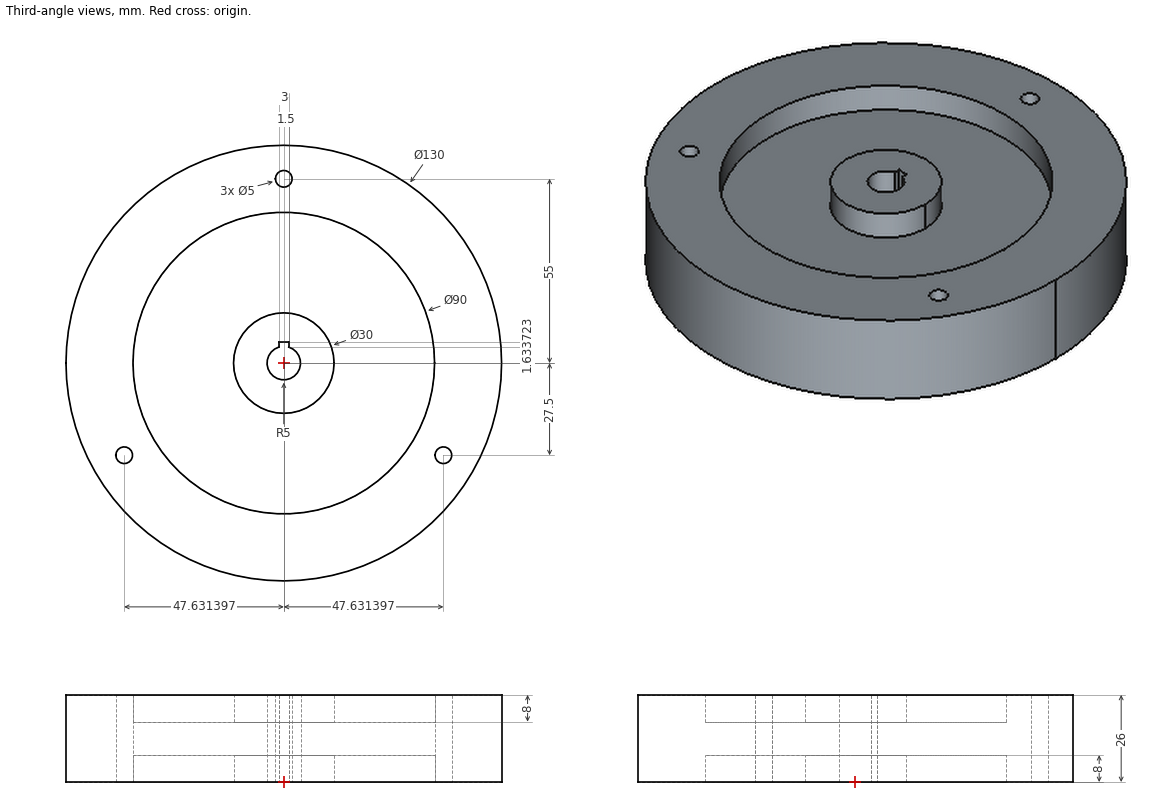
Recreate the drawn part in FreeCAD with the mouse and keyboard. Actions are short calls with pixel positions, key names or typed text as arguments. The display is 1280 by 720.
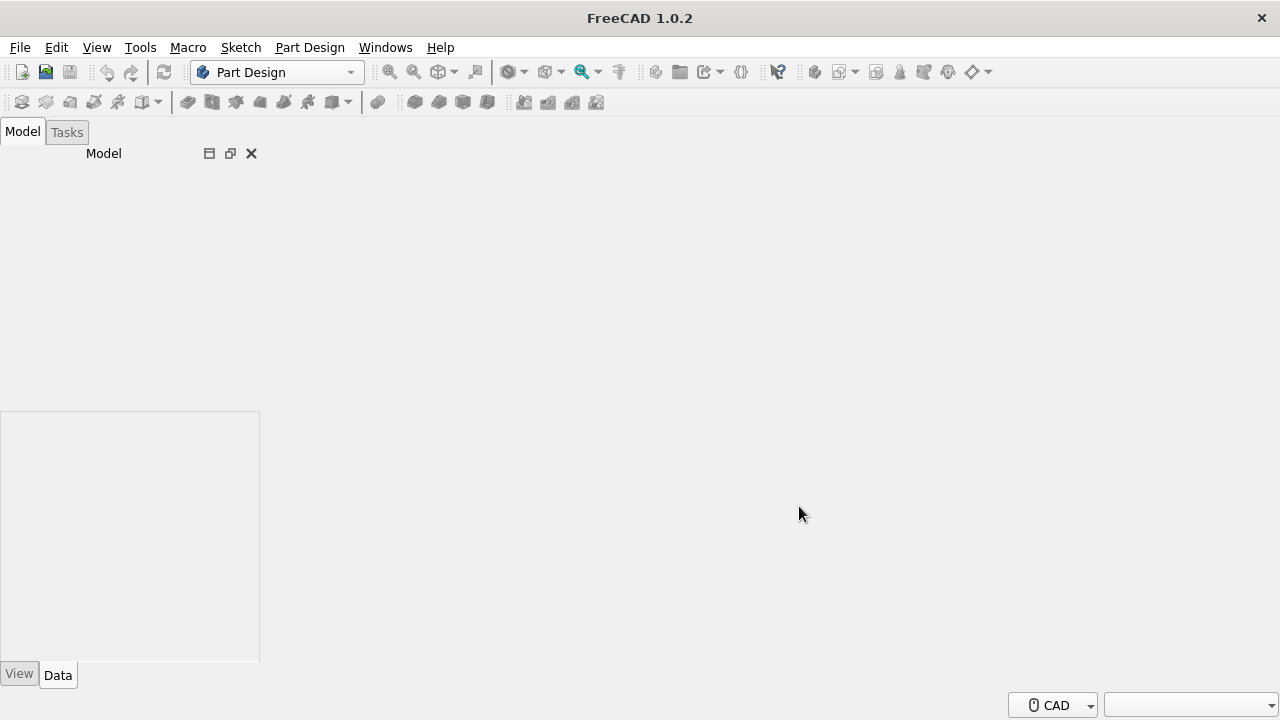
key(ctrl+n)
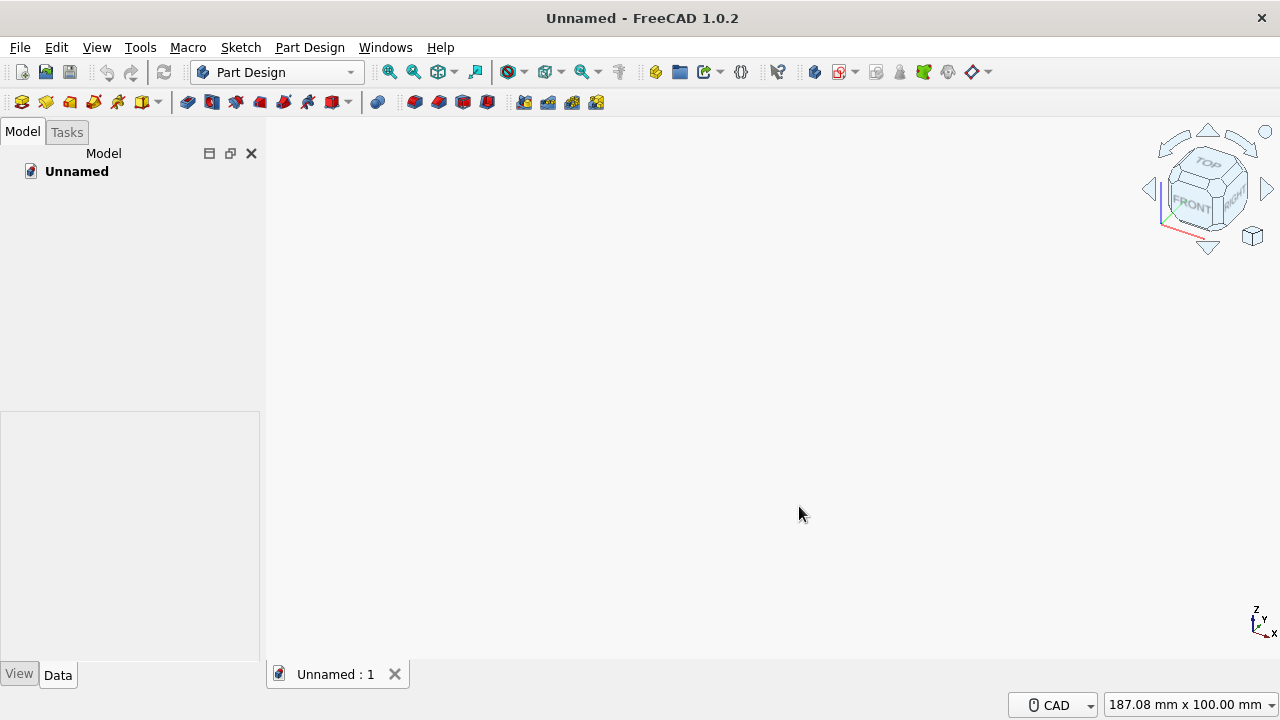
click(840, 72)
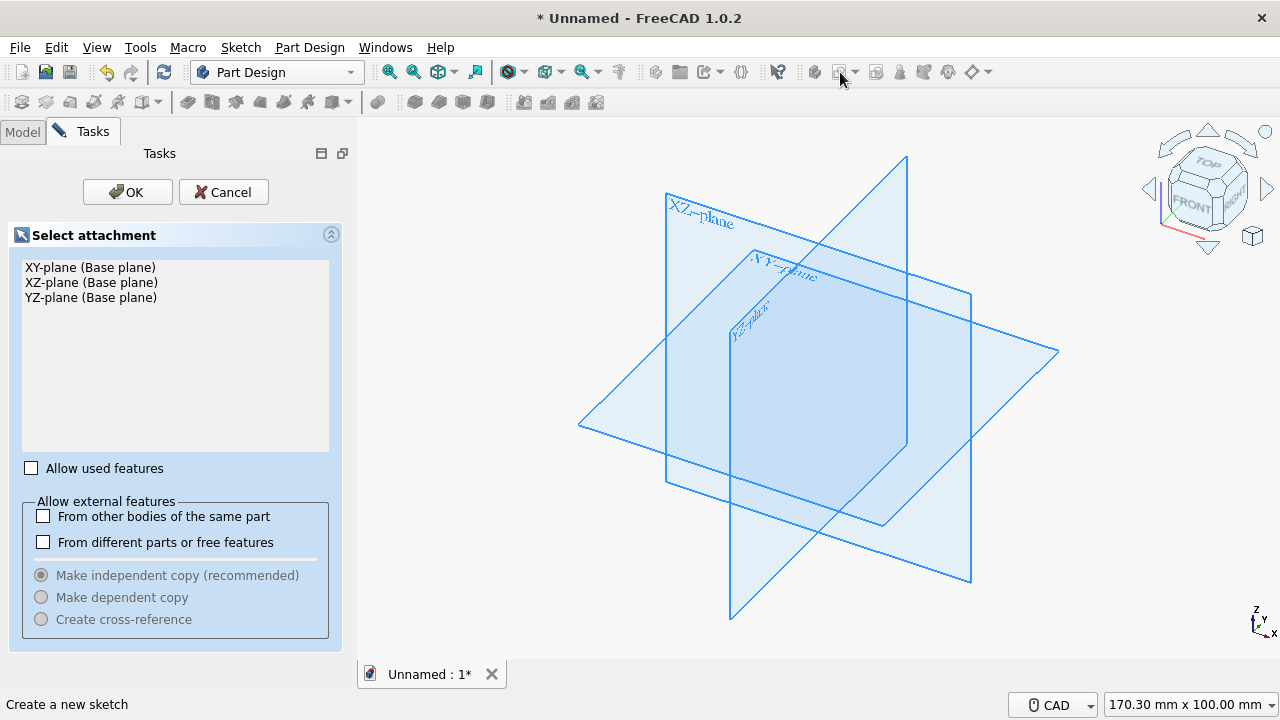
click(82, 268)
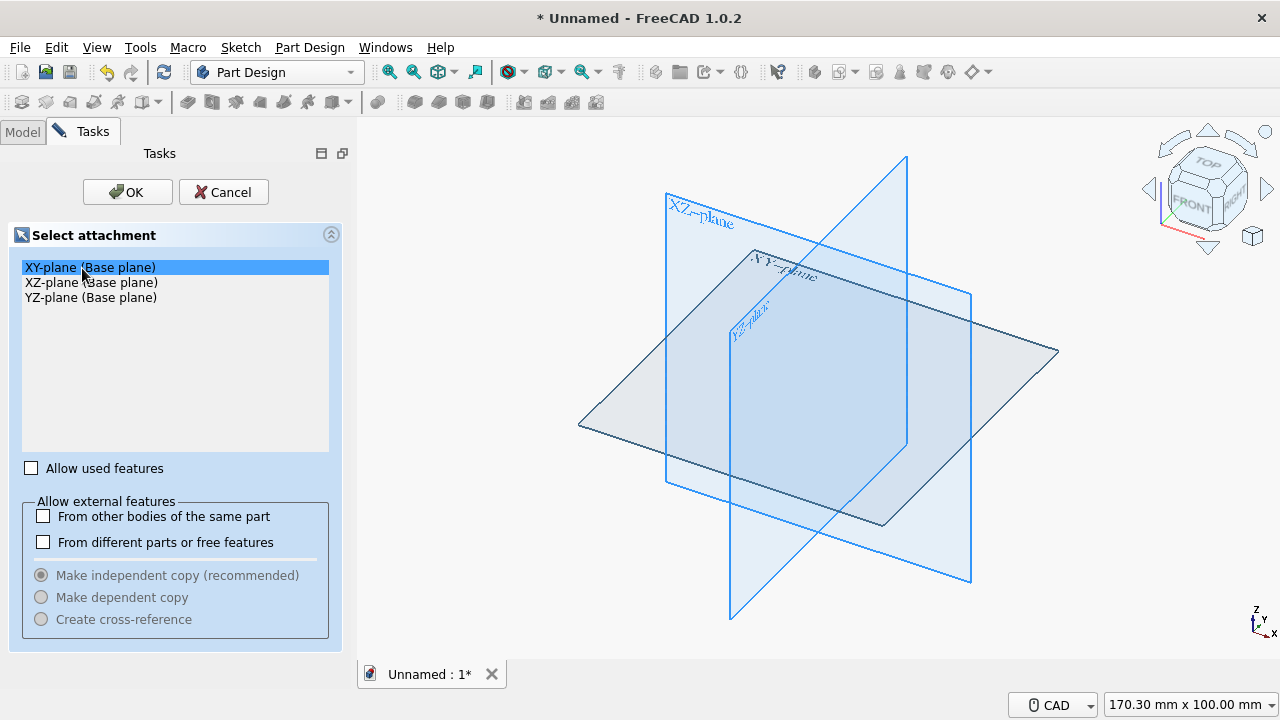
click(128, 192)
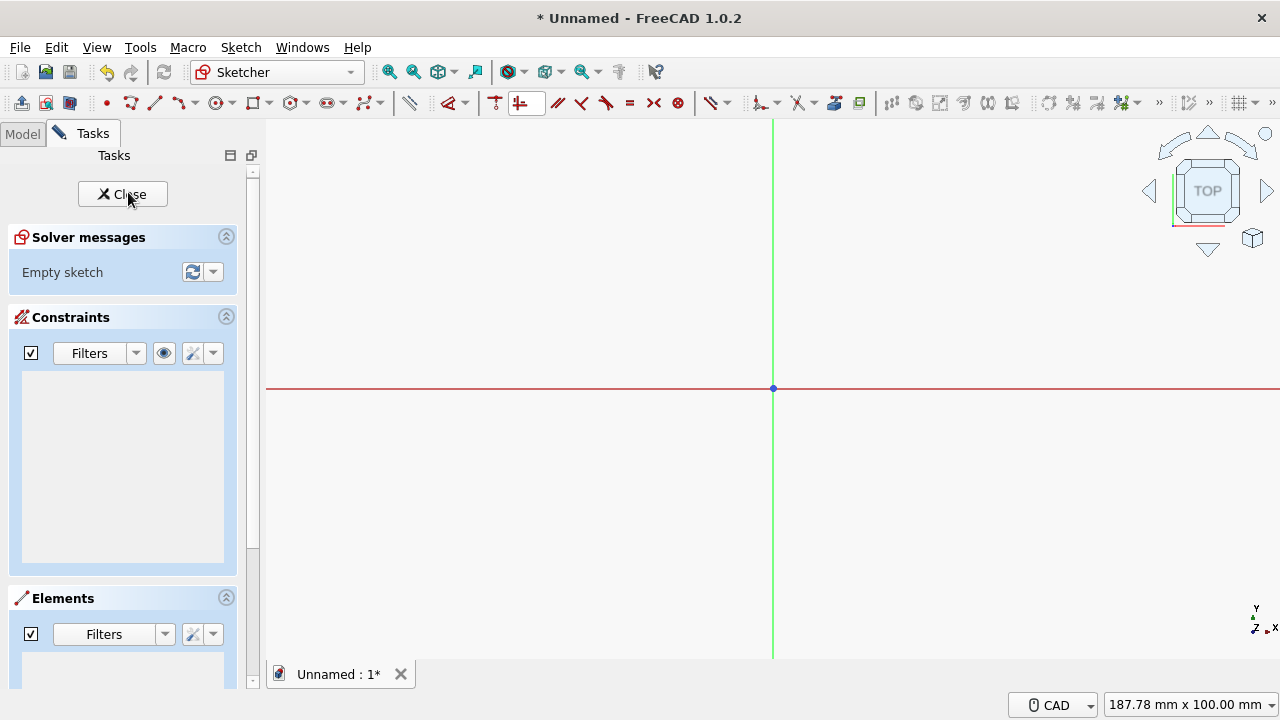
scroll(649, 389, down, 4)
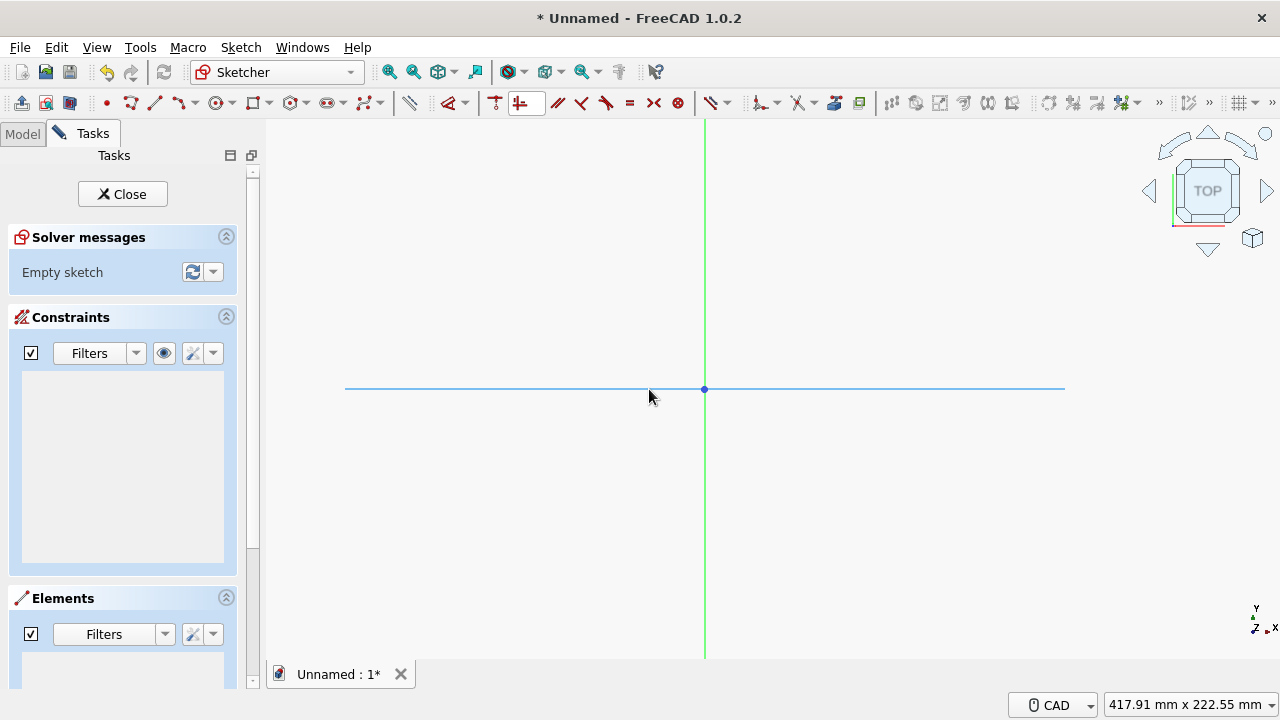
key(g)
key(c)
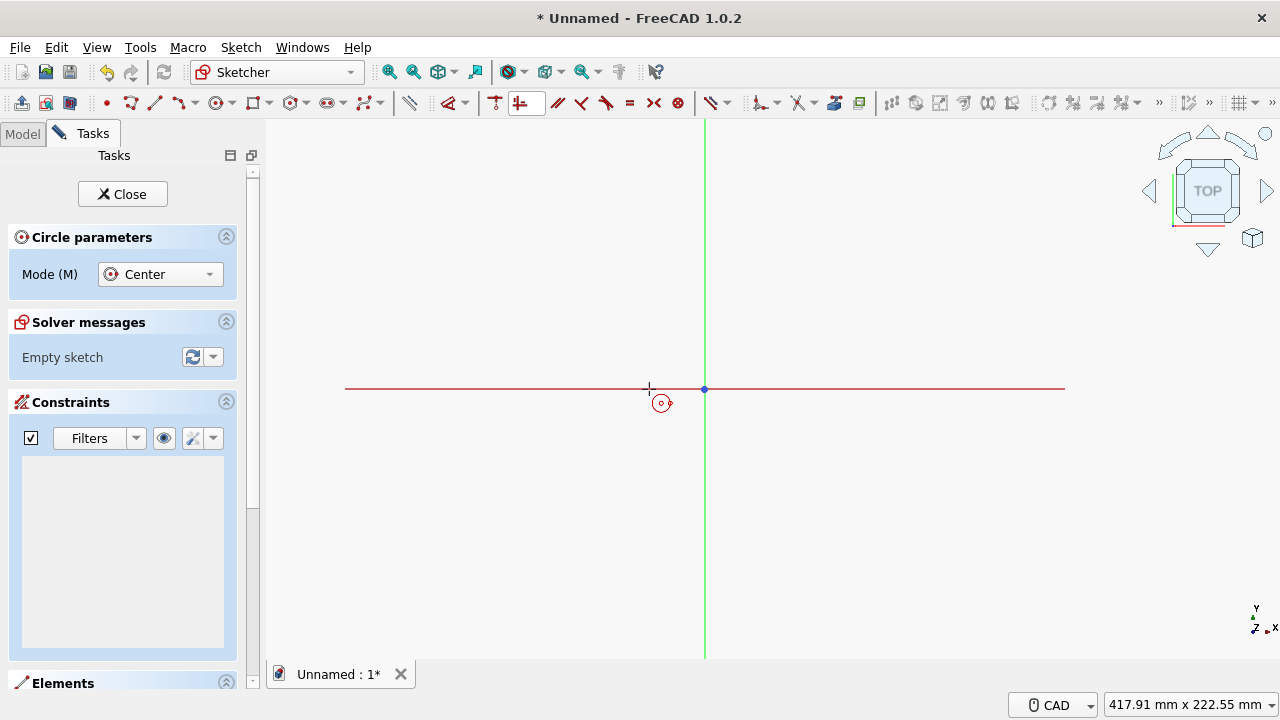
click(705, 389)
click(816, 278)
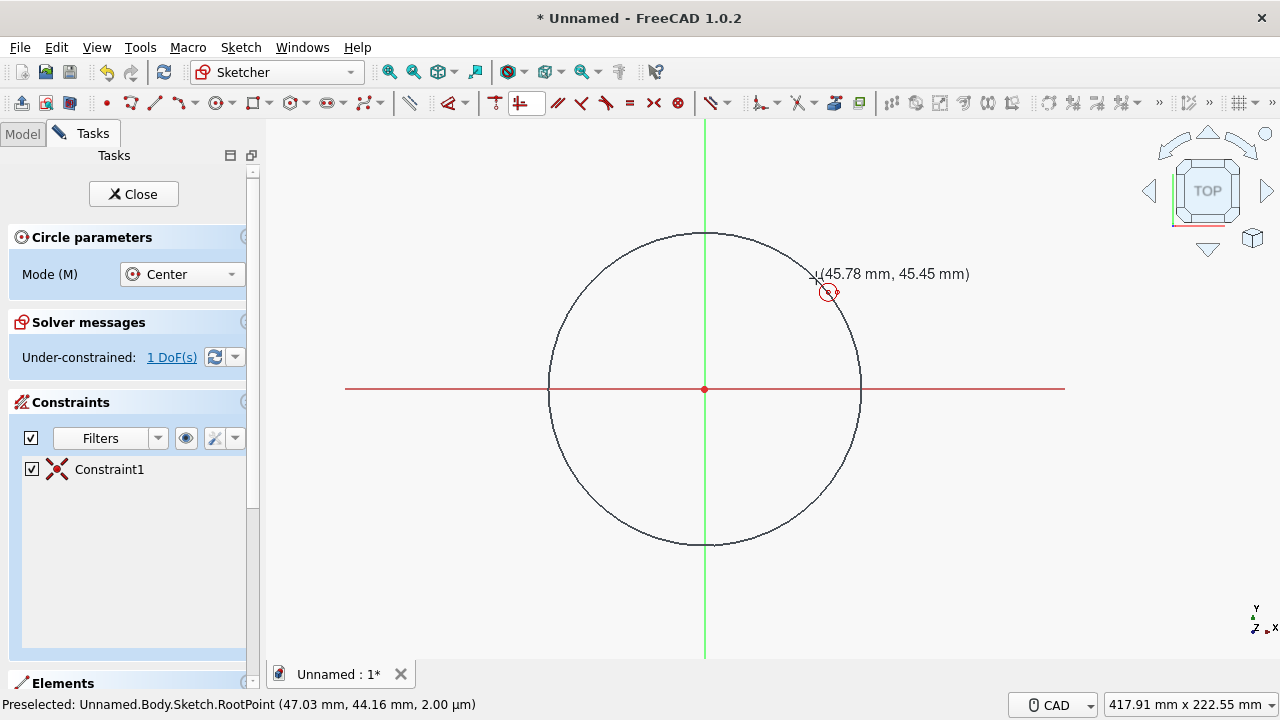
scroll(705, 256, up, 7)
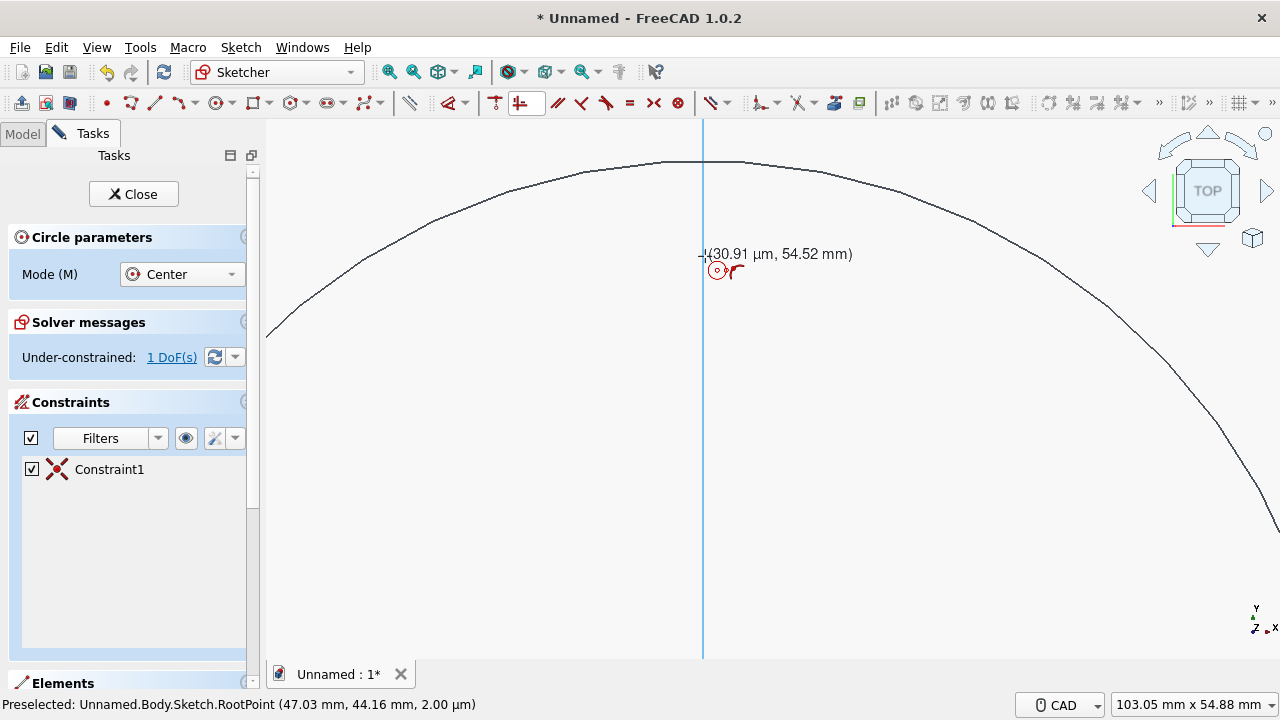
scroll(705, 256, down, 7)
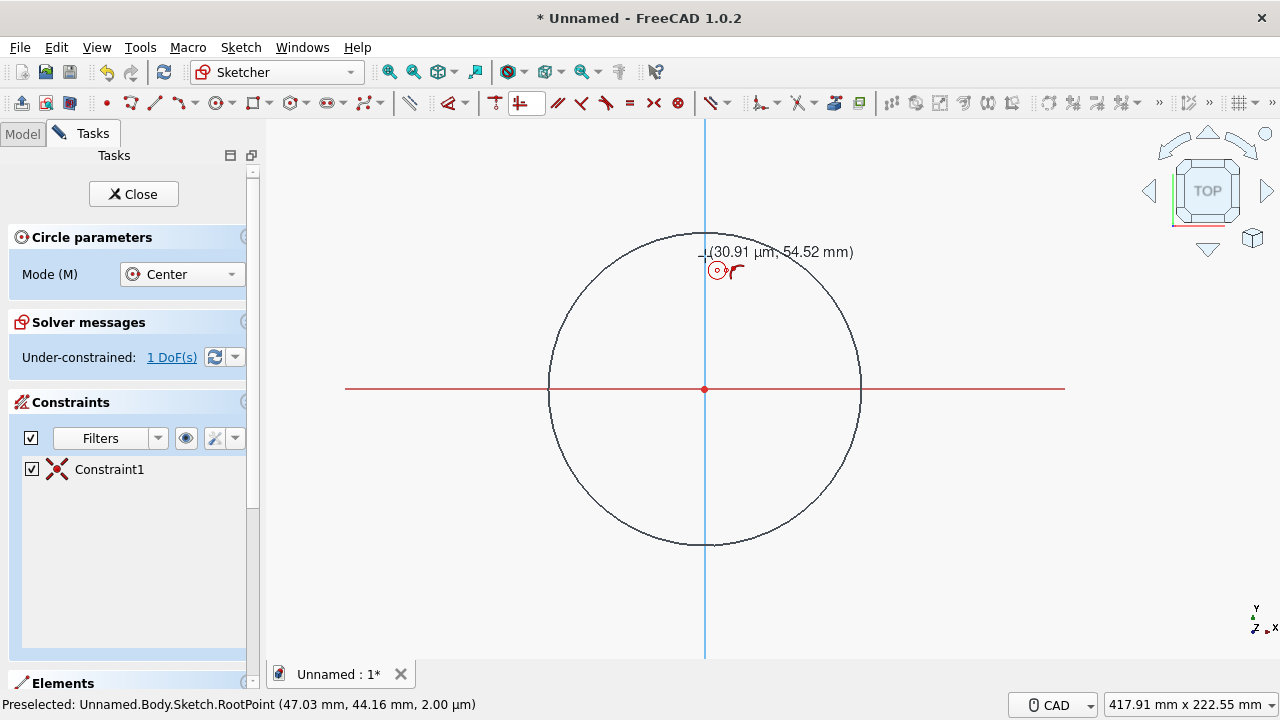
click(705, 256)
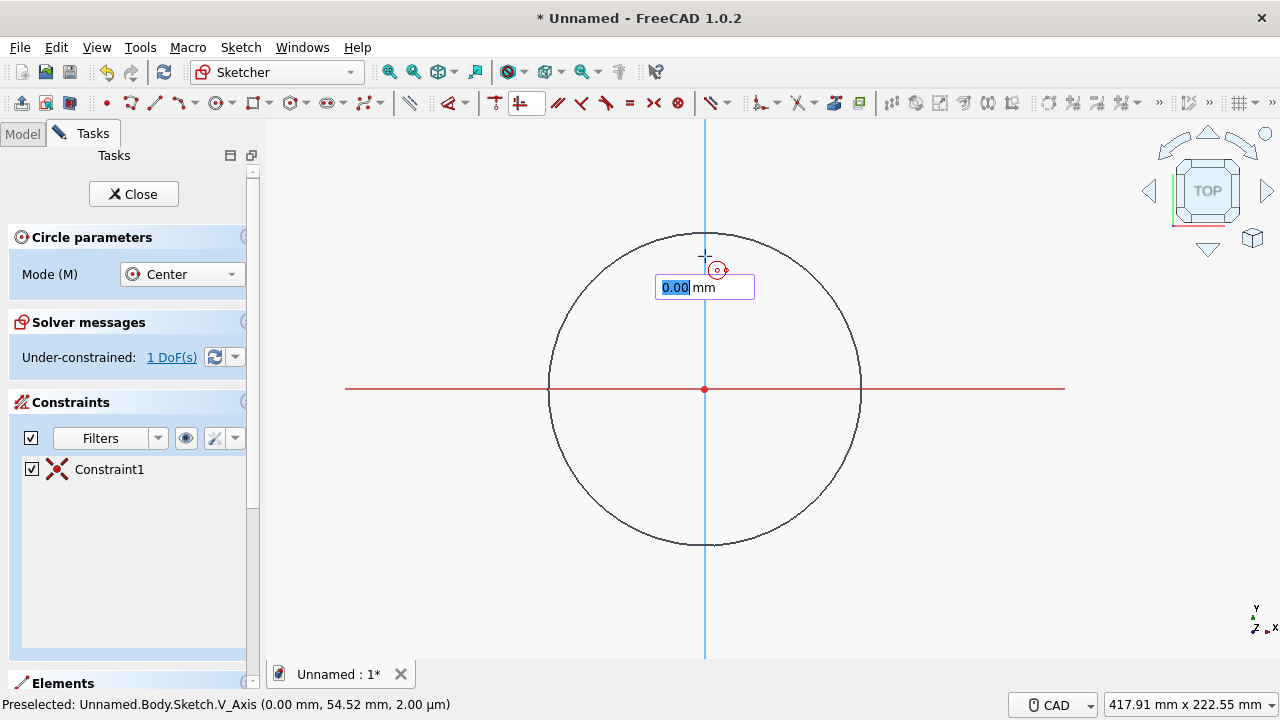
scroll(711, 254, up, 6)